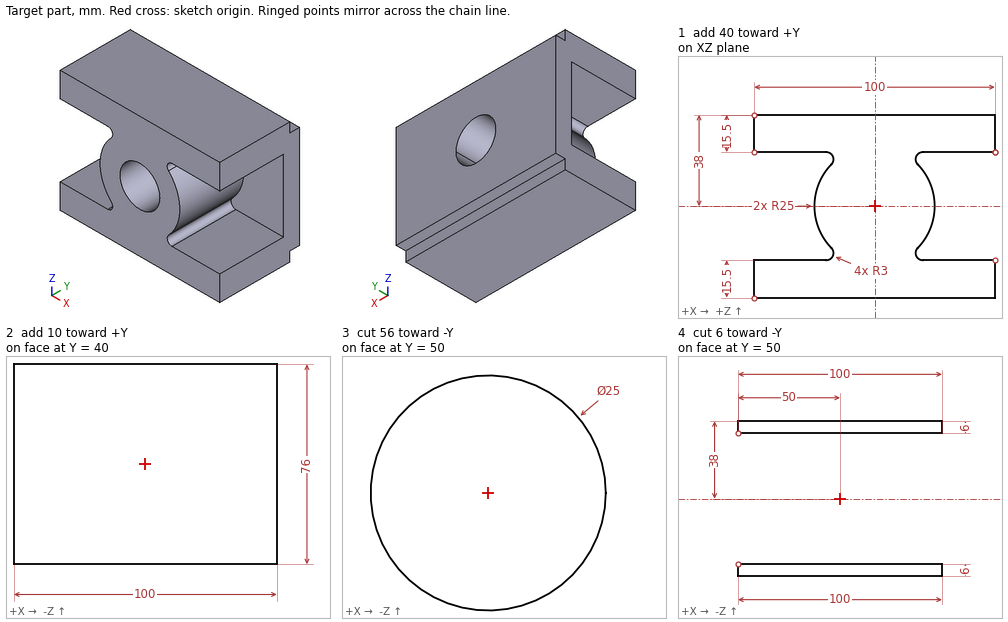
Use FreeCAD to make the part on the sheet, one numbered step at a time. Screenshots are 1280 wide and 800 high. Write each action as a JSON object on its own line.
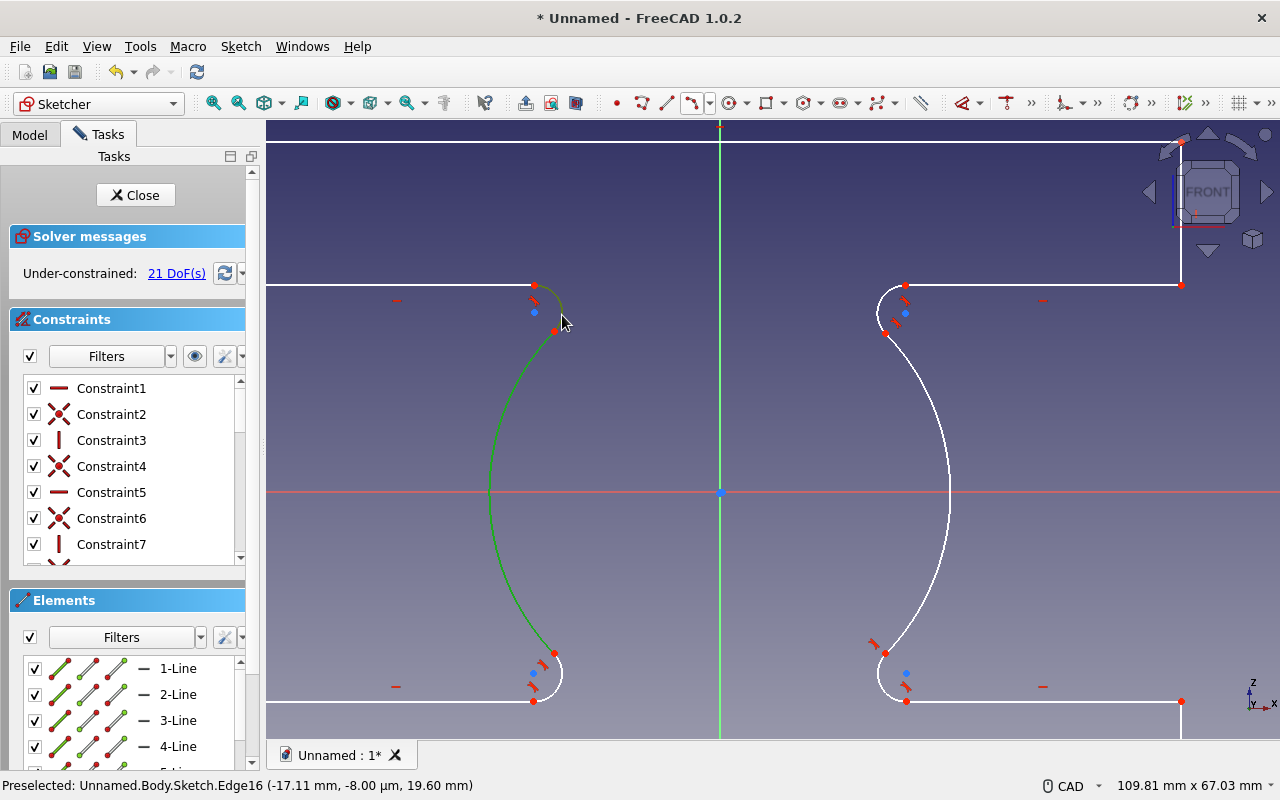
{"action": "key", "text": "t"}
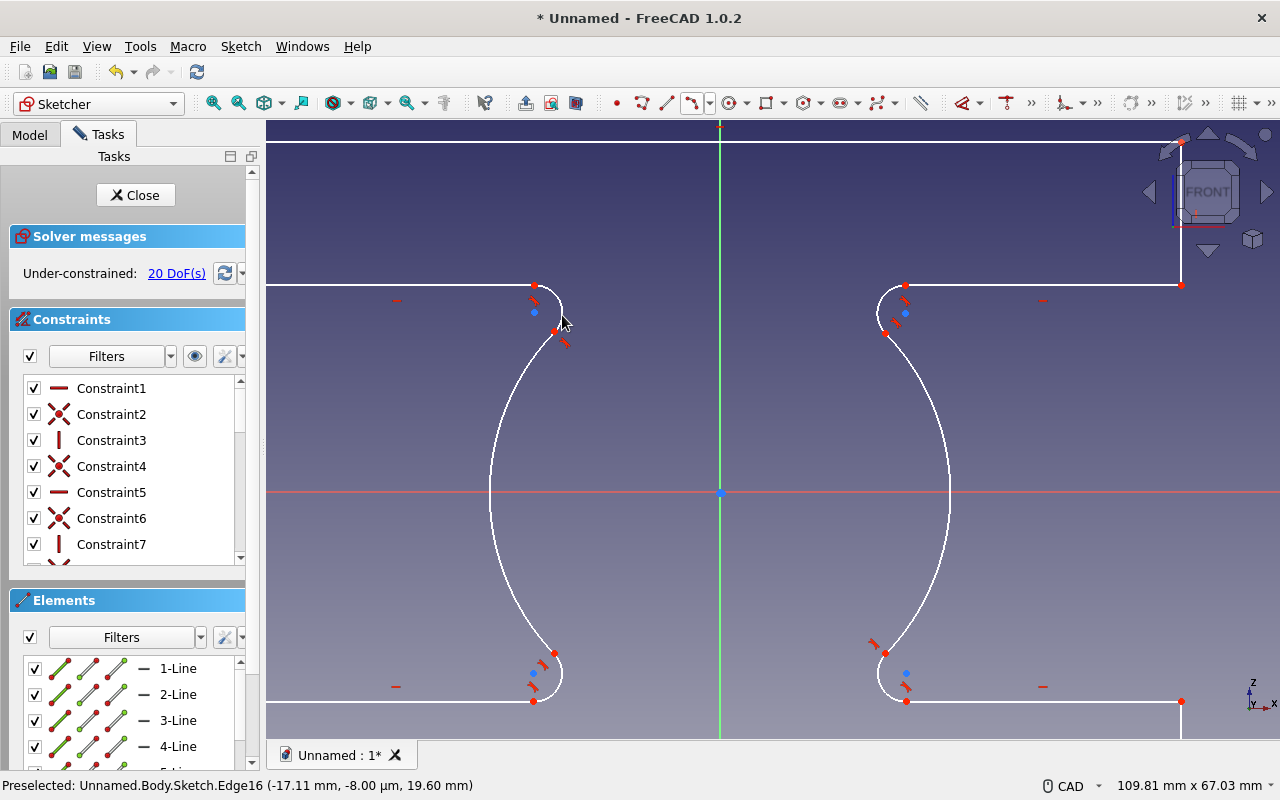
{"action": "left_click", "coordinate": [940, 563]}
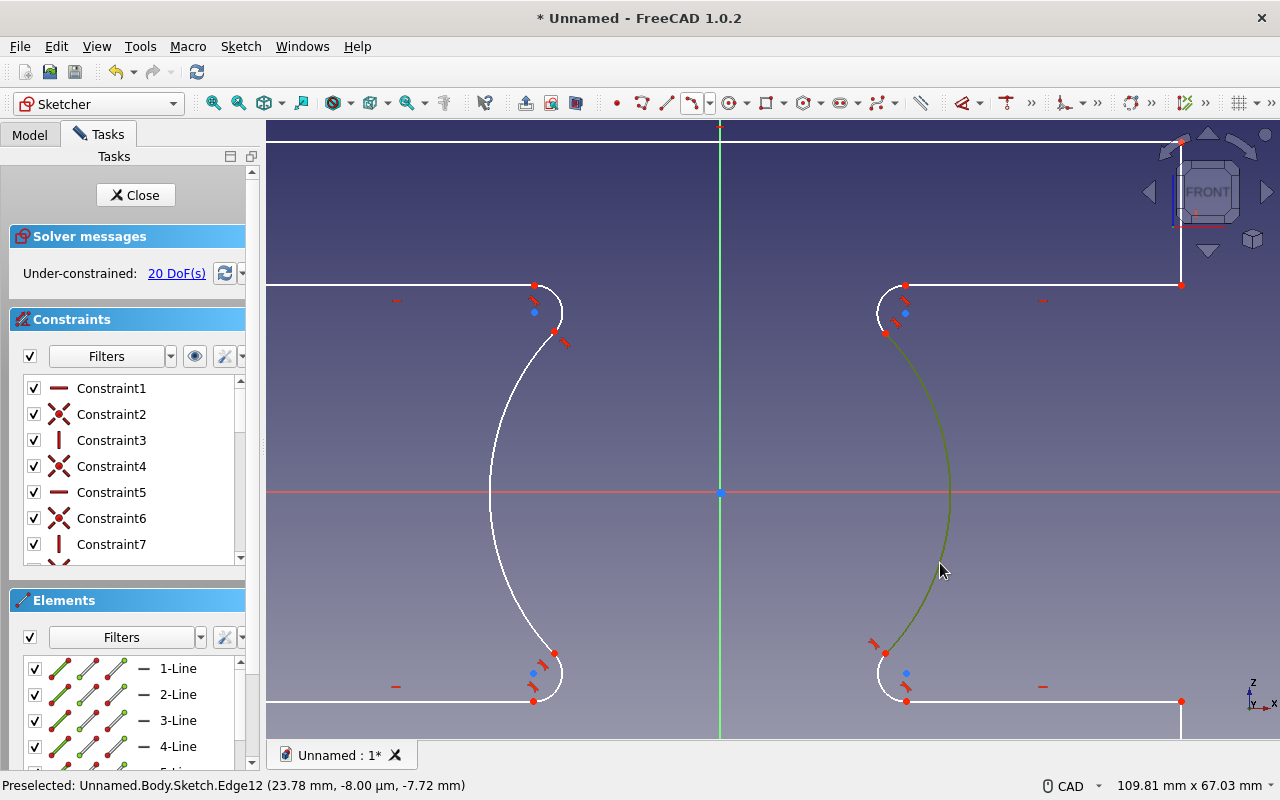
{"action": "left_click", "coordinate": [501, 423]}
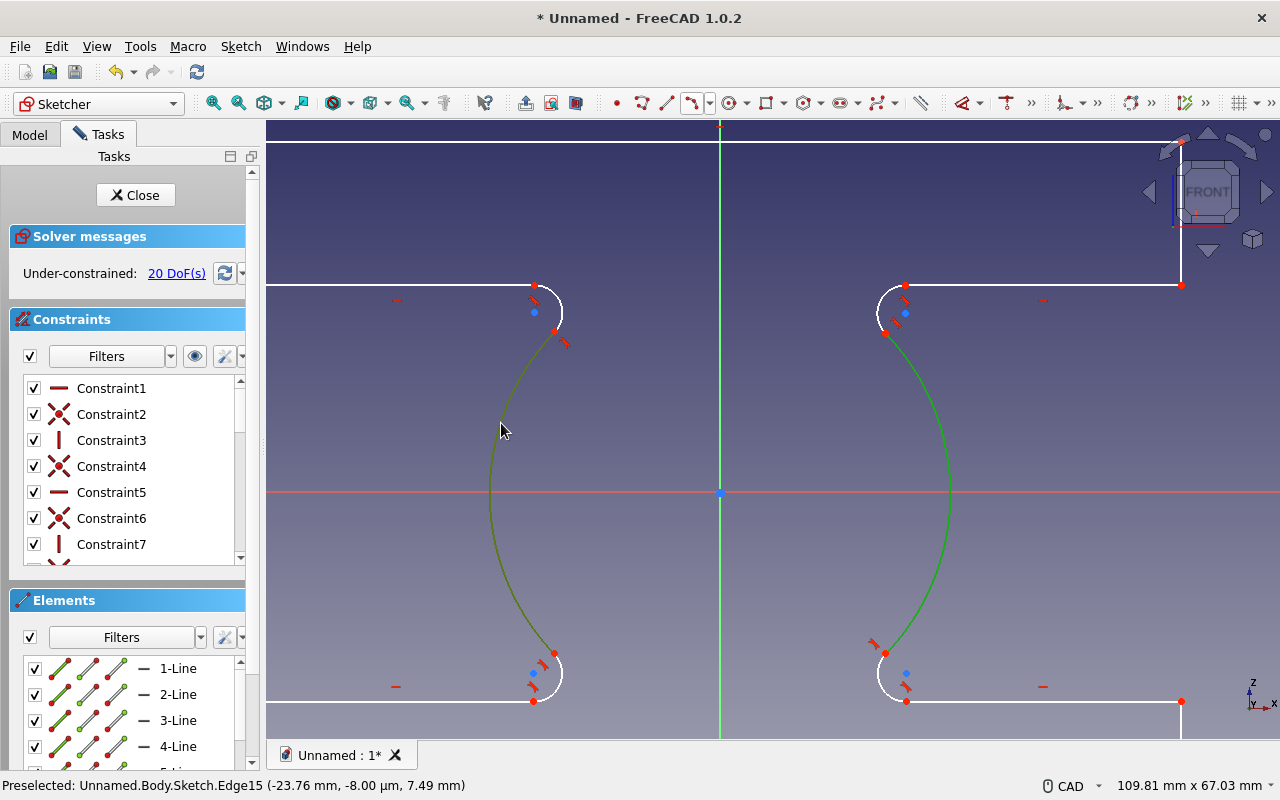
{"action": "left_click", "coordinate": [1006, 104]}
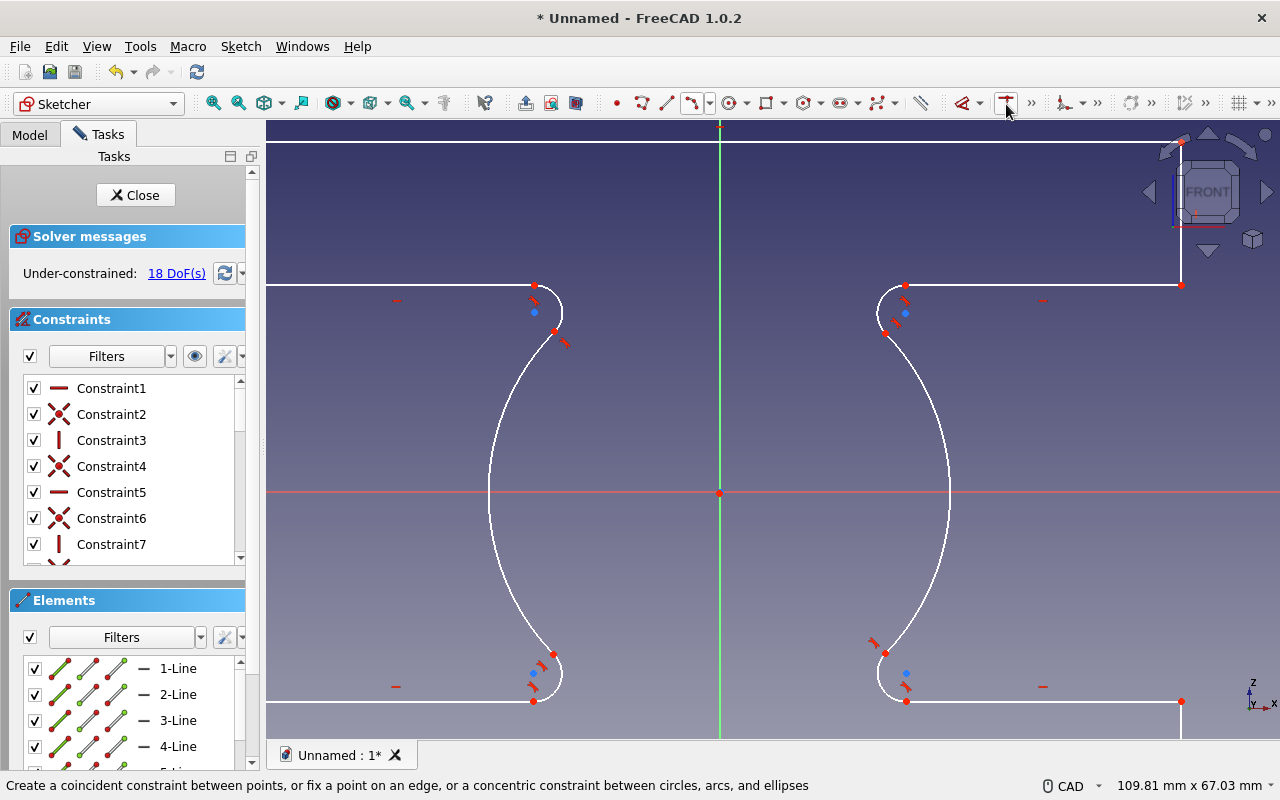
{"action": "scroll", "coordinate": [720, 493], "scroll_direction": "up", "scroll_amount": 2}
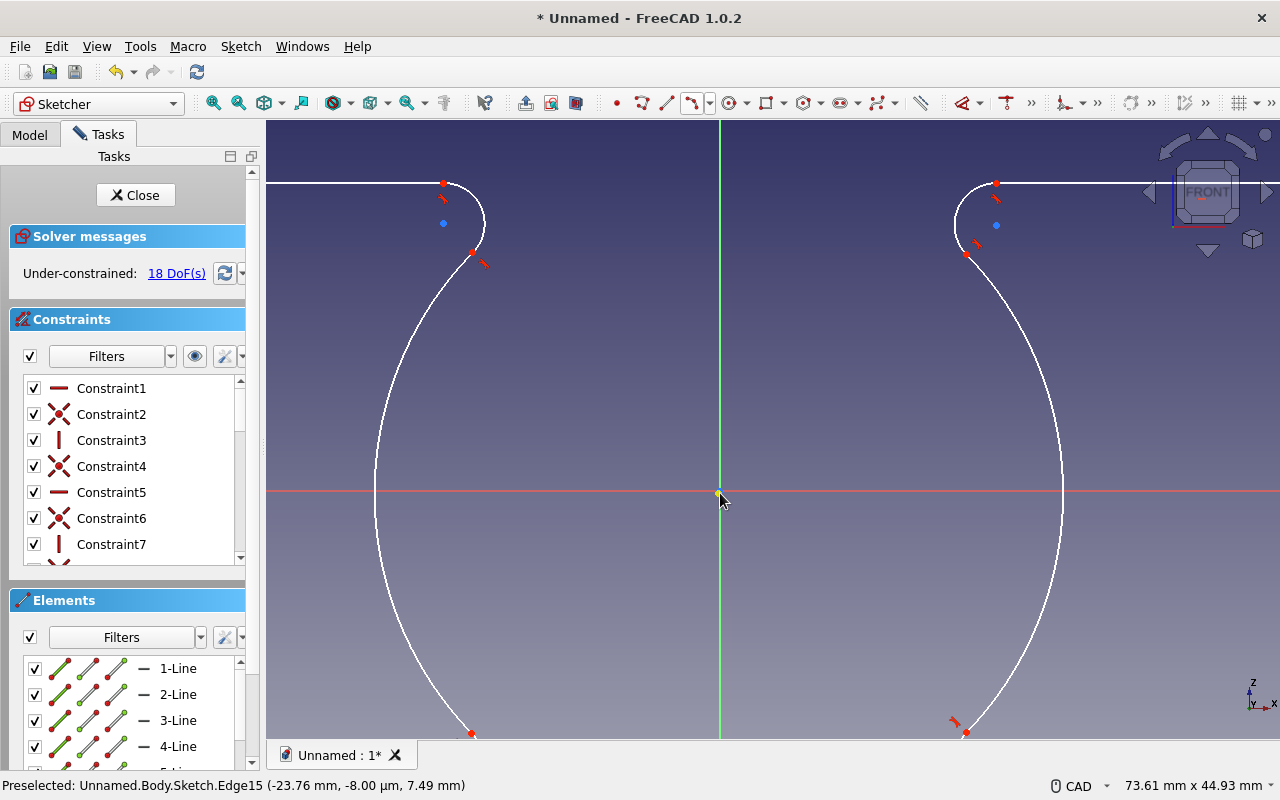
{"action": "left_click_drag", "start_coordinate": [709, 481], "coordinate": [730, 503]}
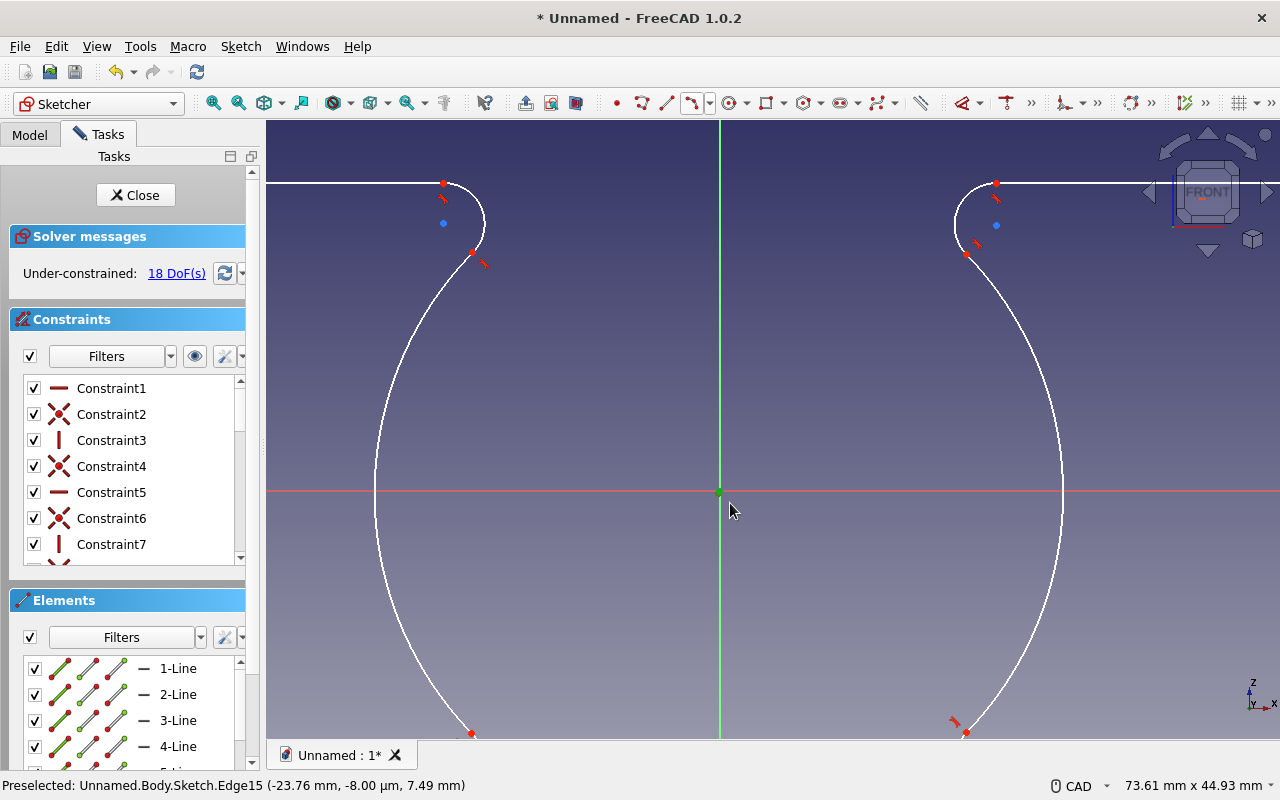
{"action": "left_click", "coordinate": [1006, 104]}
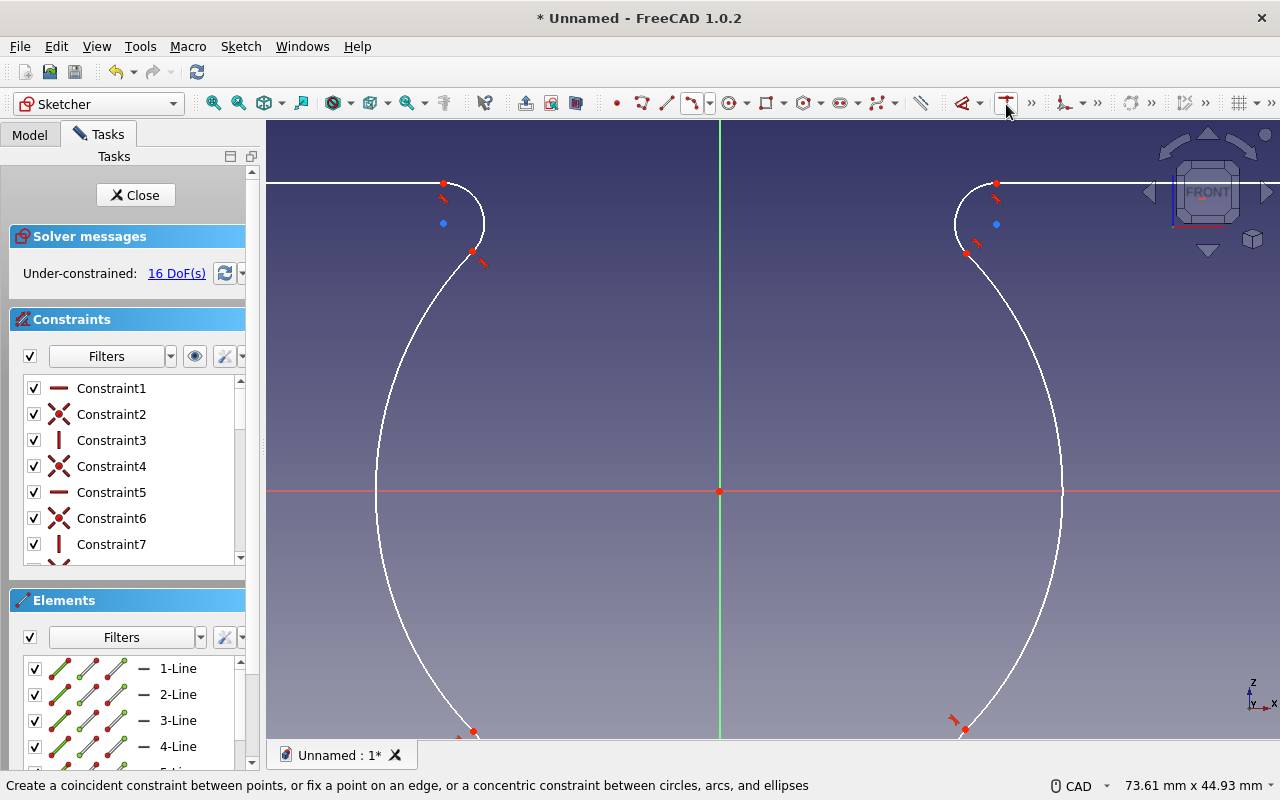
{"action": "left_click", "coordinate": [970, 193]}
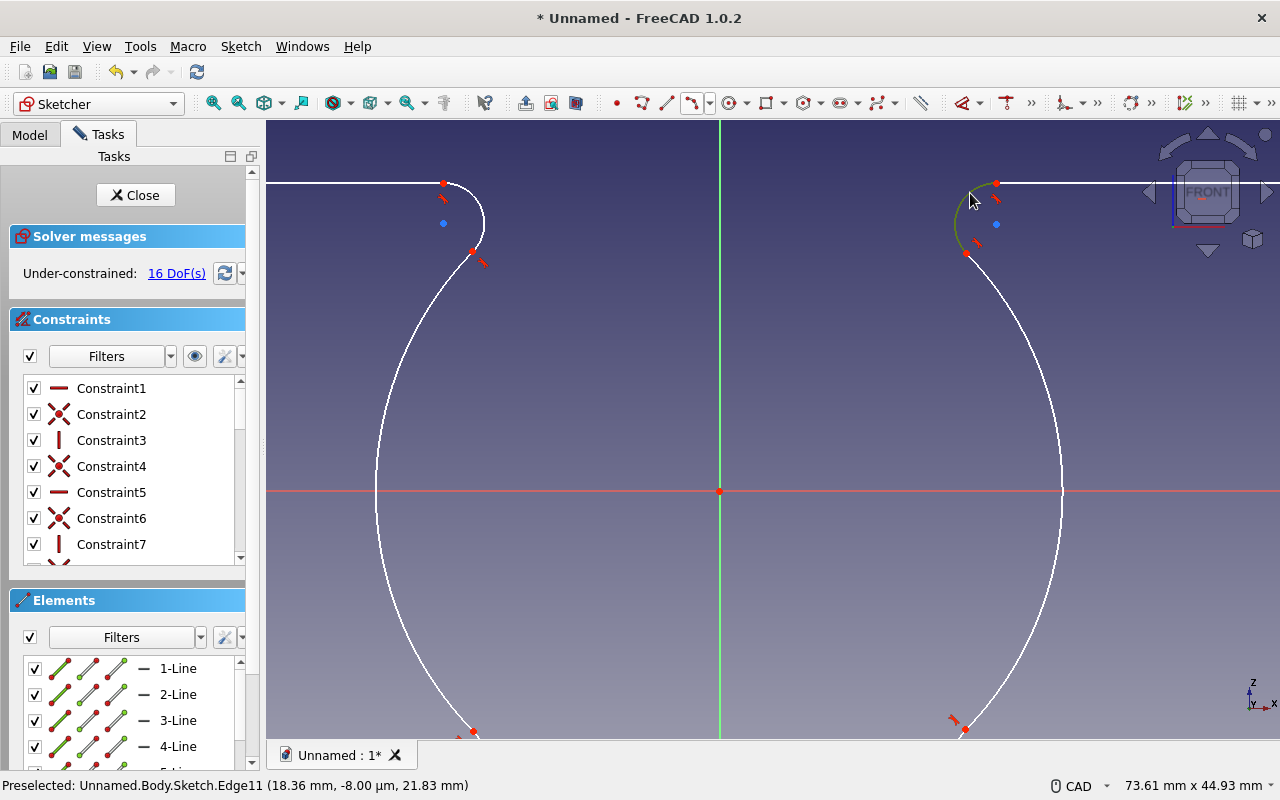
{"action": "scroll", "coordinate": [696, 394], "scroll_direction": "down", "scroll_amount": 5}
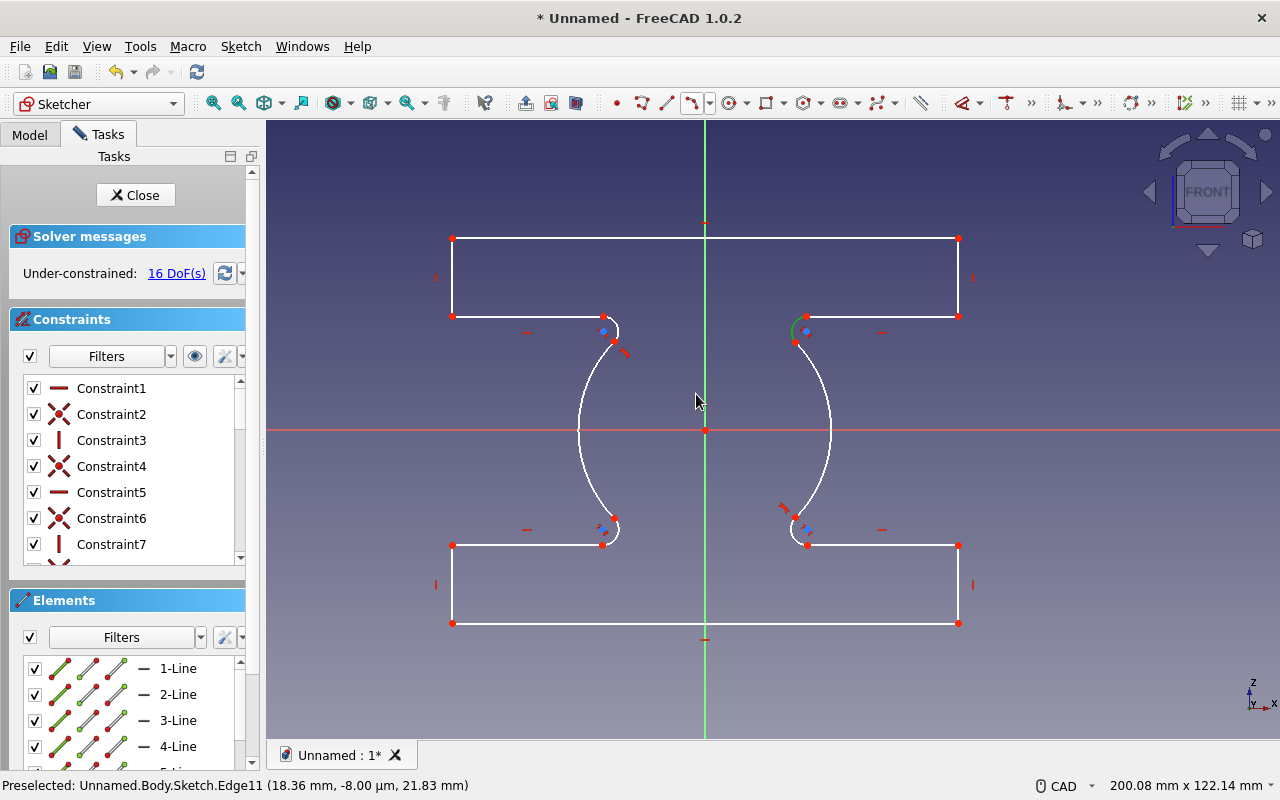
{"action": "scroll", "coordinate": [791, 528], "scroll_direction": "up", "scroll_amount": 2}